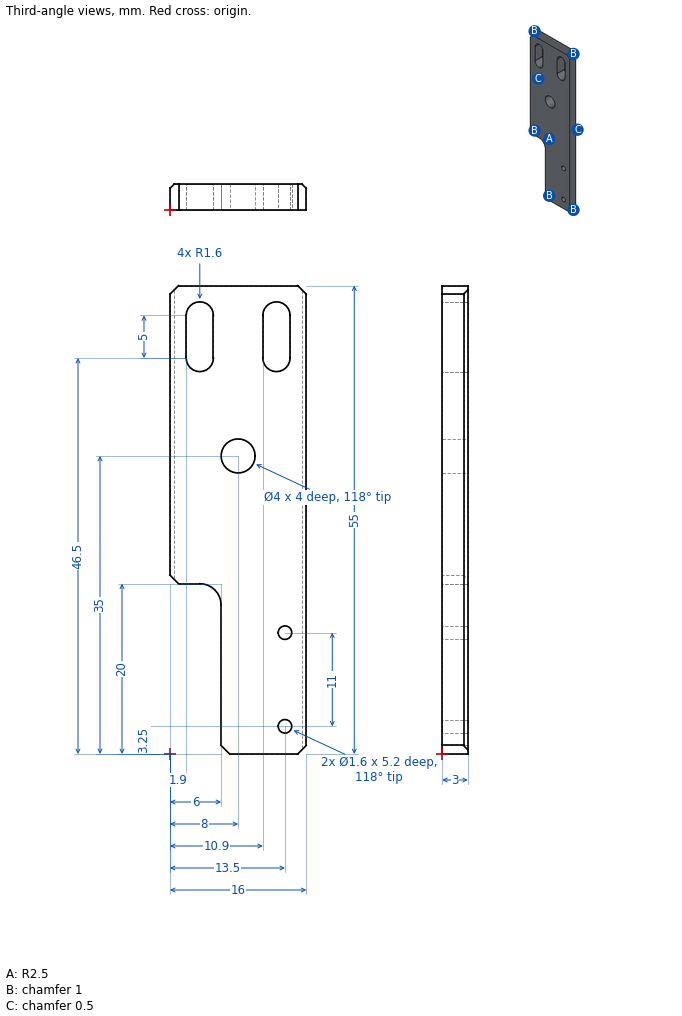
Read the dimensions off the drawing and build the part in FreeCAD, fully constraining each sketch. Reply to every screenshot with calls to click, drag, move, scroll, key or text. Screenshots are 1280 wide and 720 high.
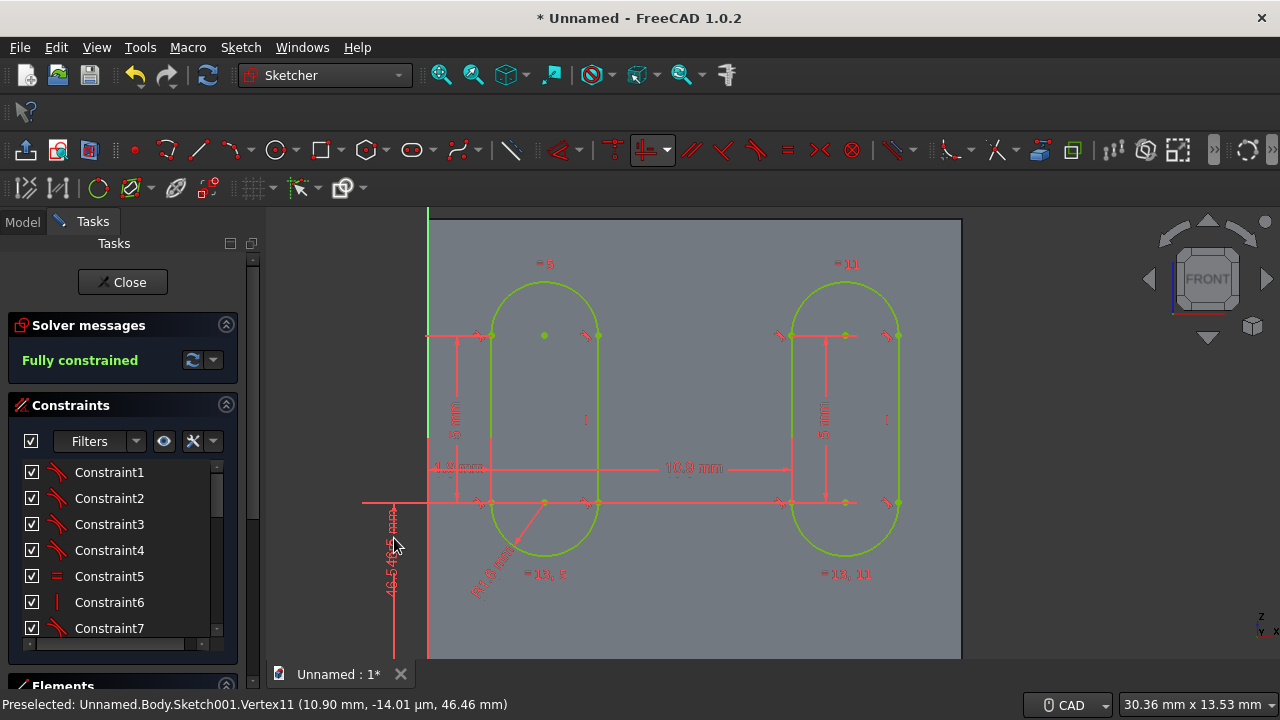
click(123, 282)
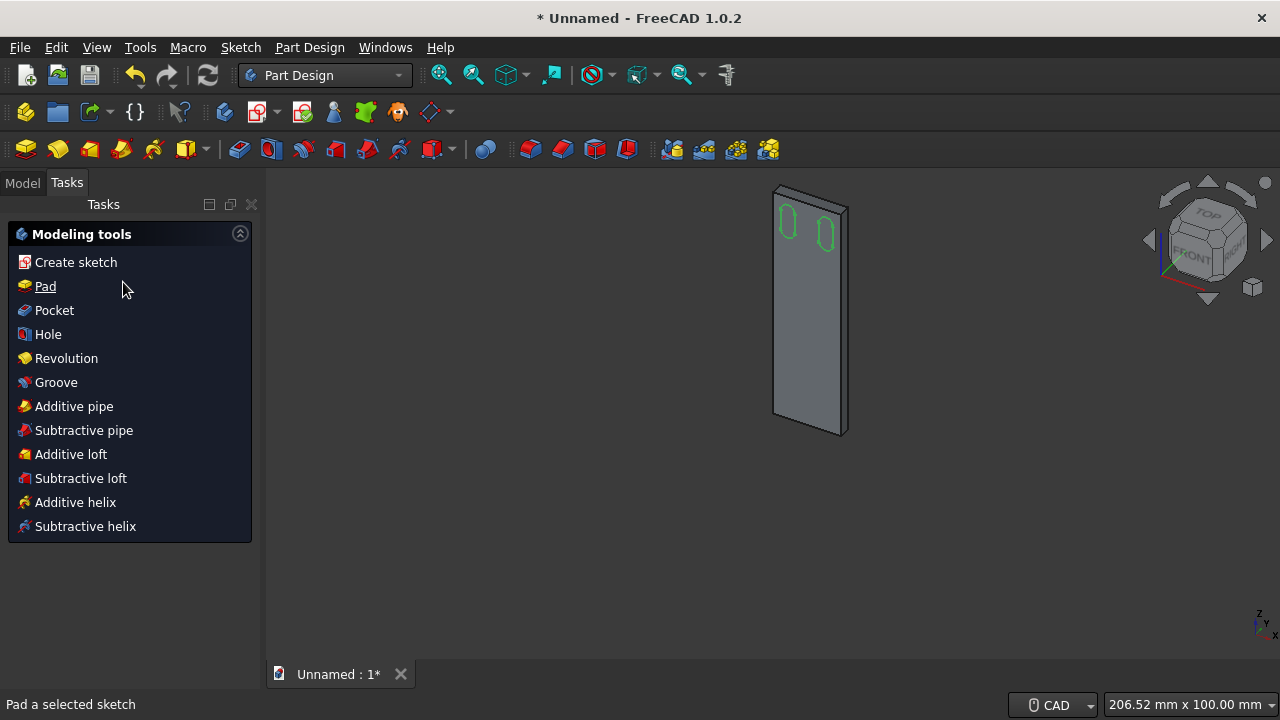
click(240, 150)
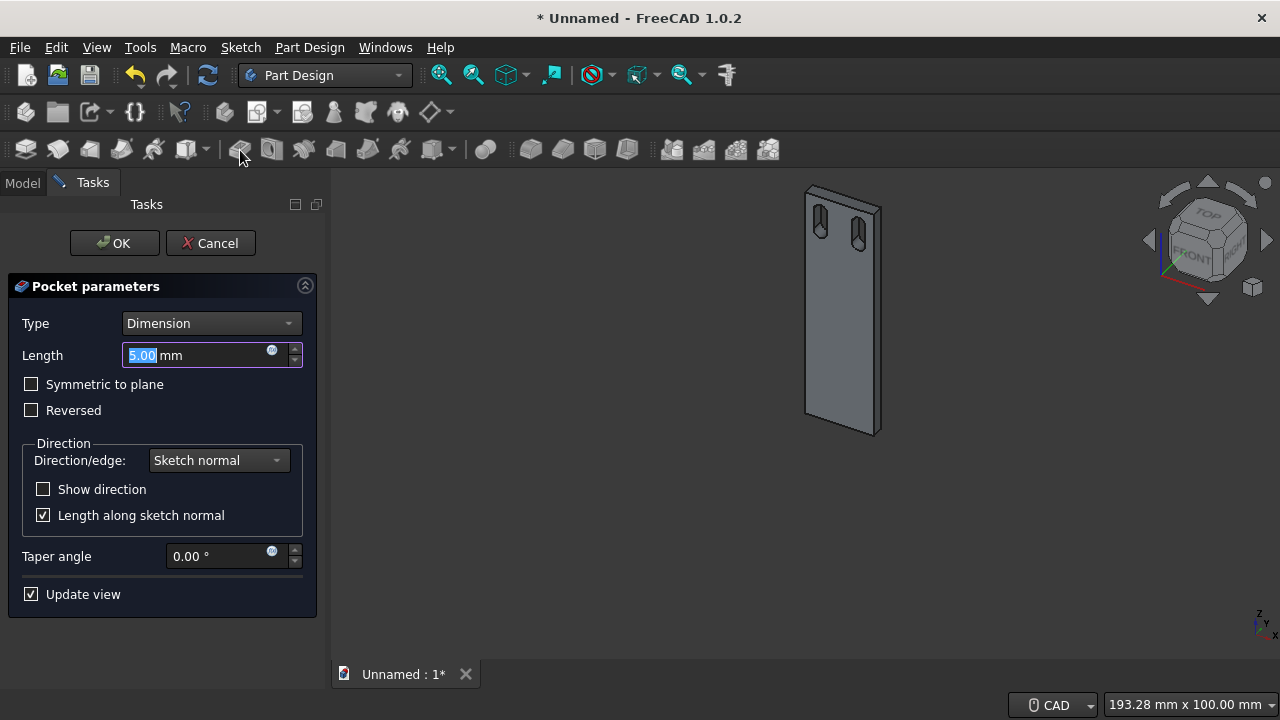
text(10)
key(Tab)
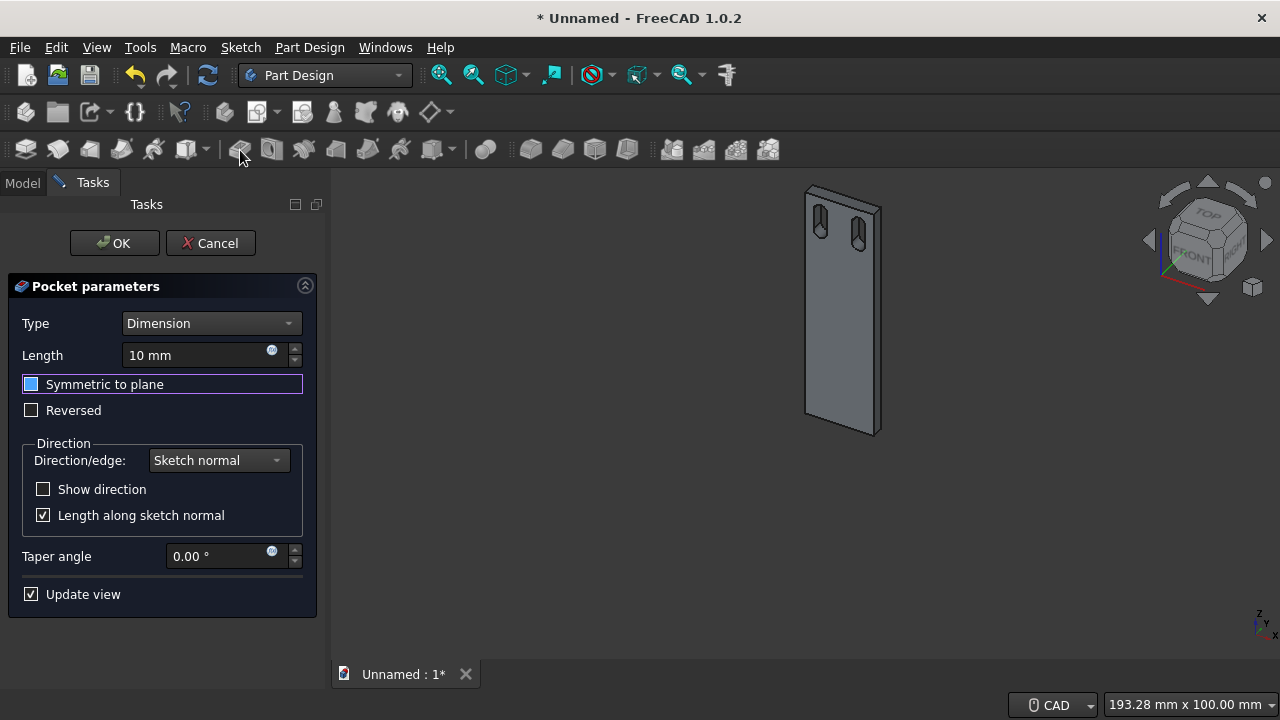
click(115, 243)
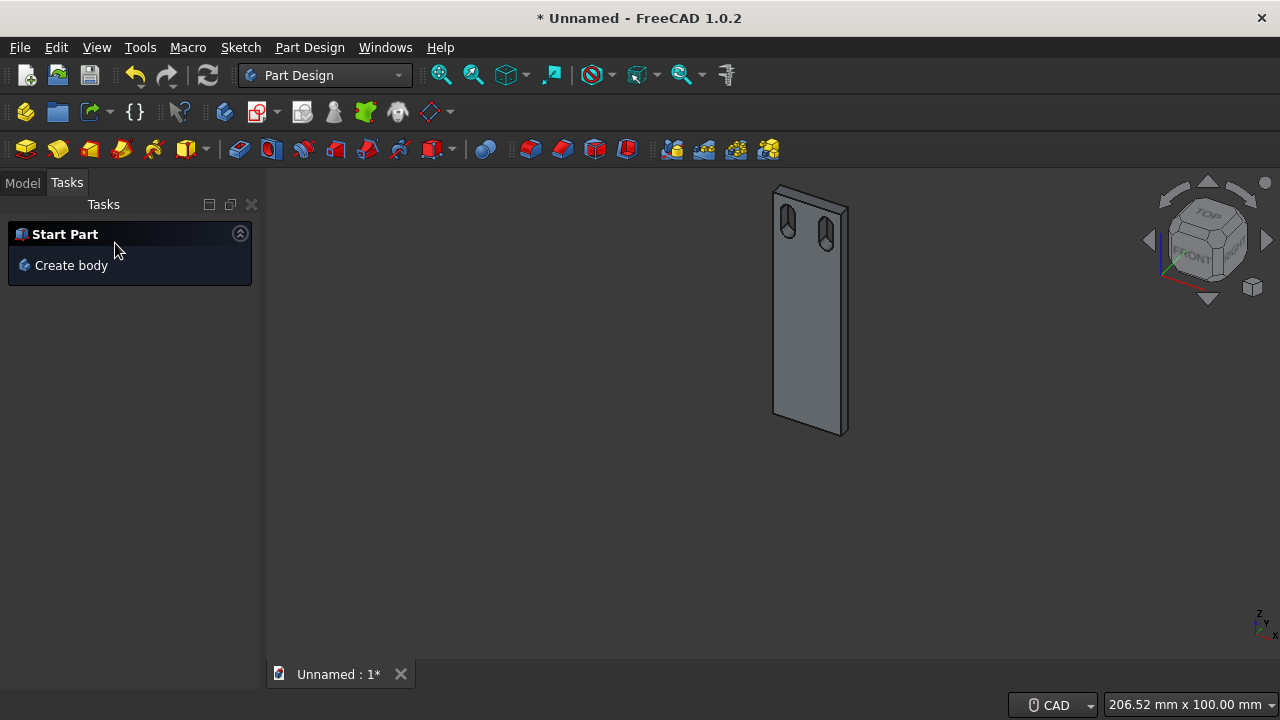
key(4)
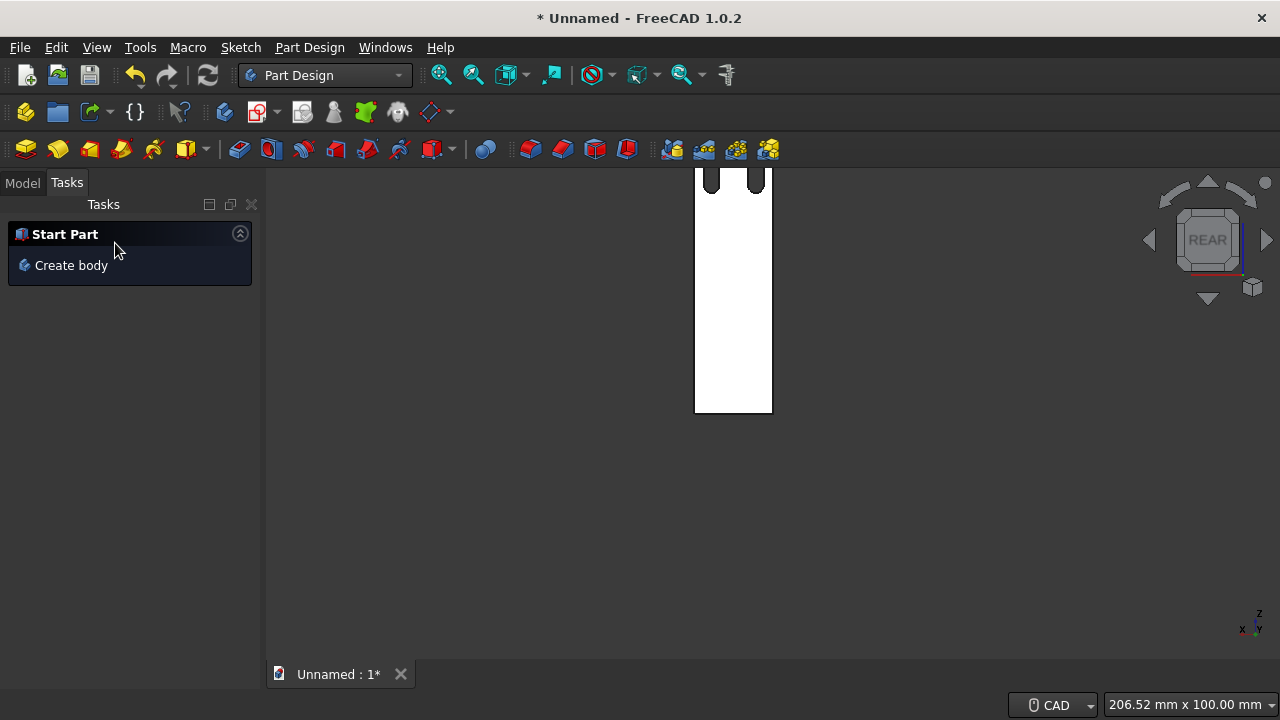
click(442, 76)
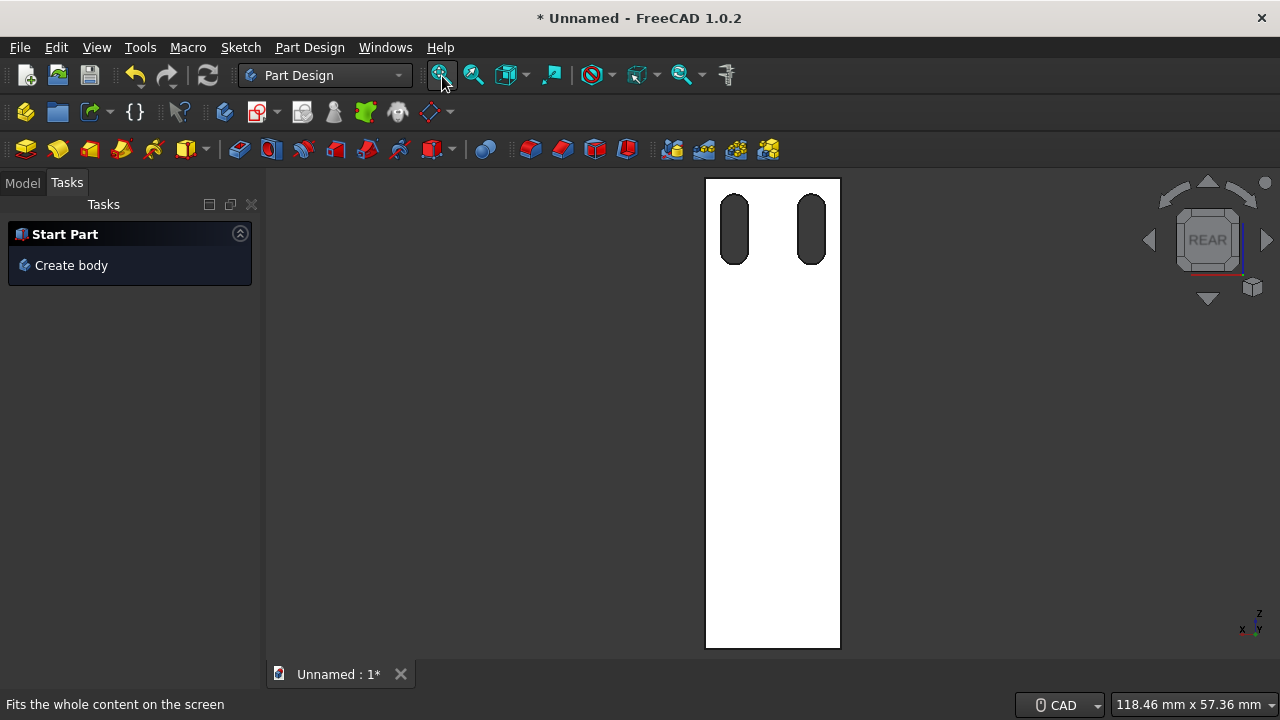
click(773, 345)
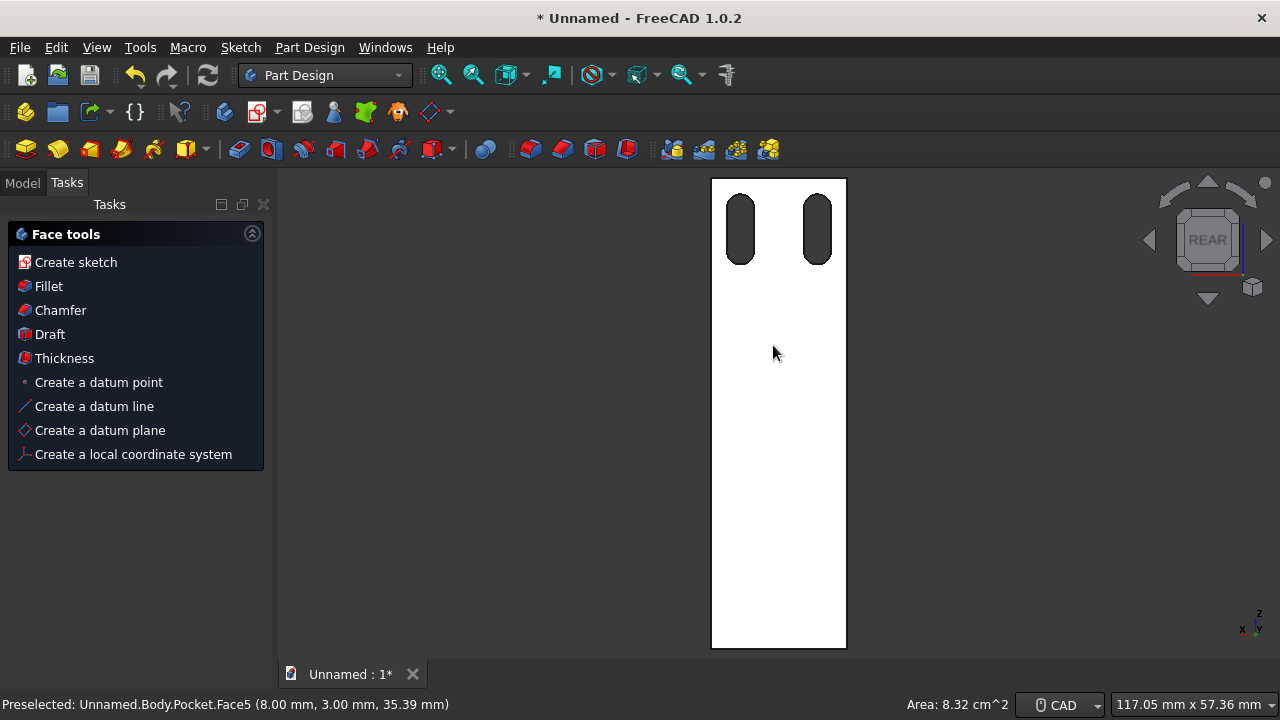
click(258, 112)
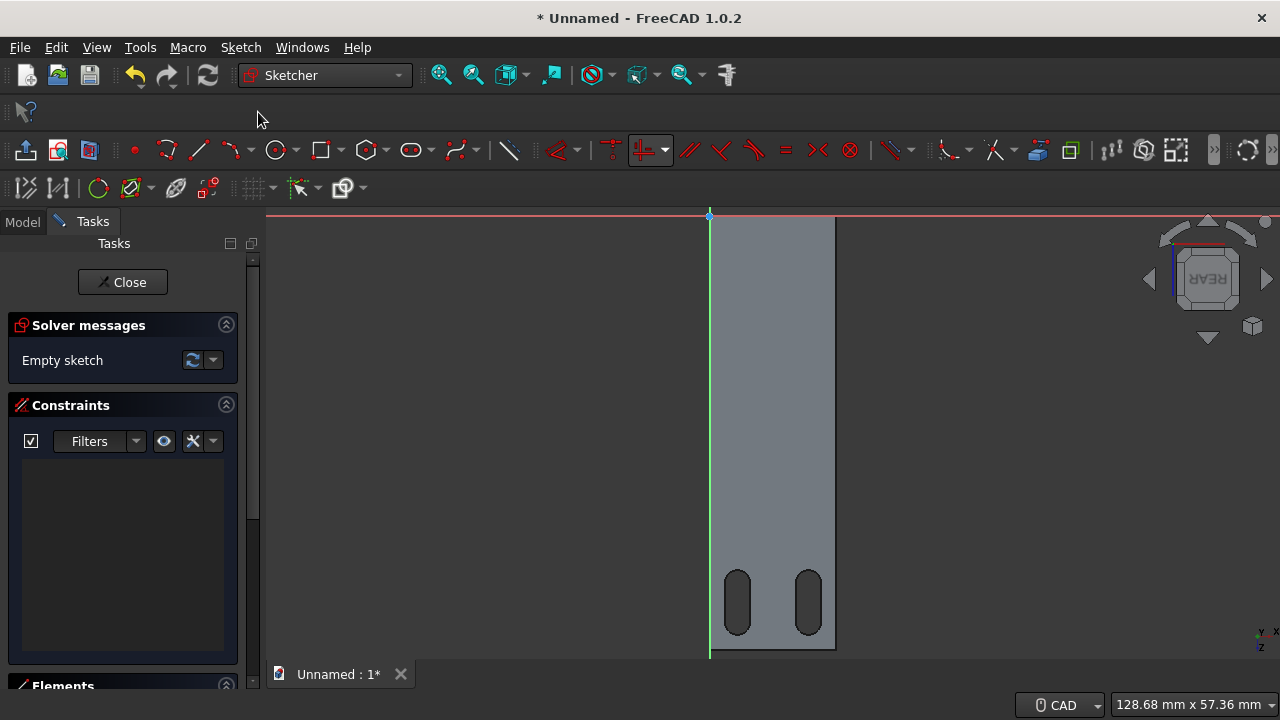
scroll(704, 433, down, 5)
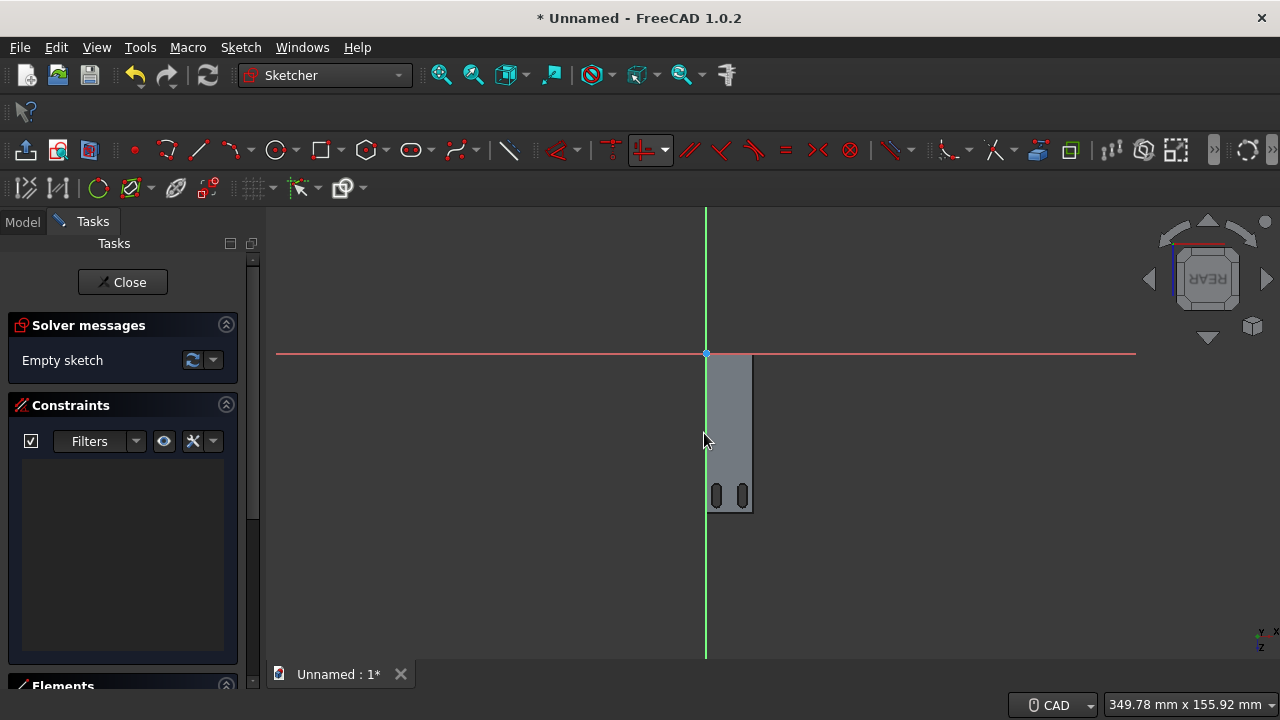
scroll(718, 370, up, 8)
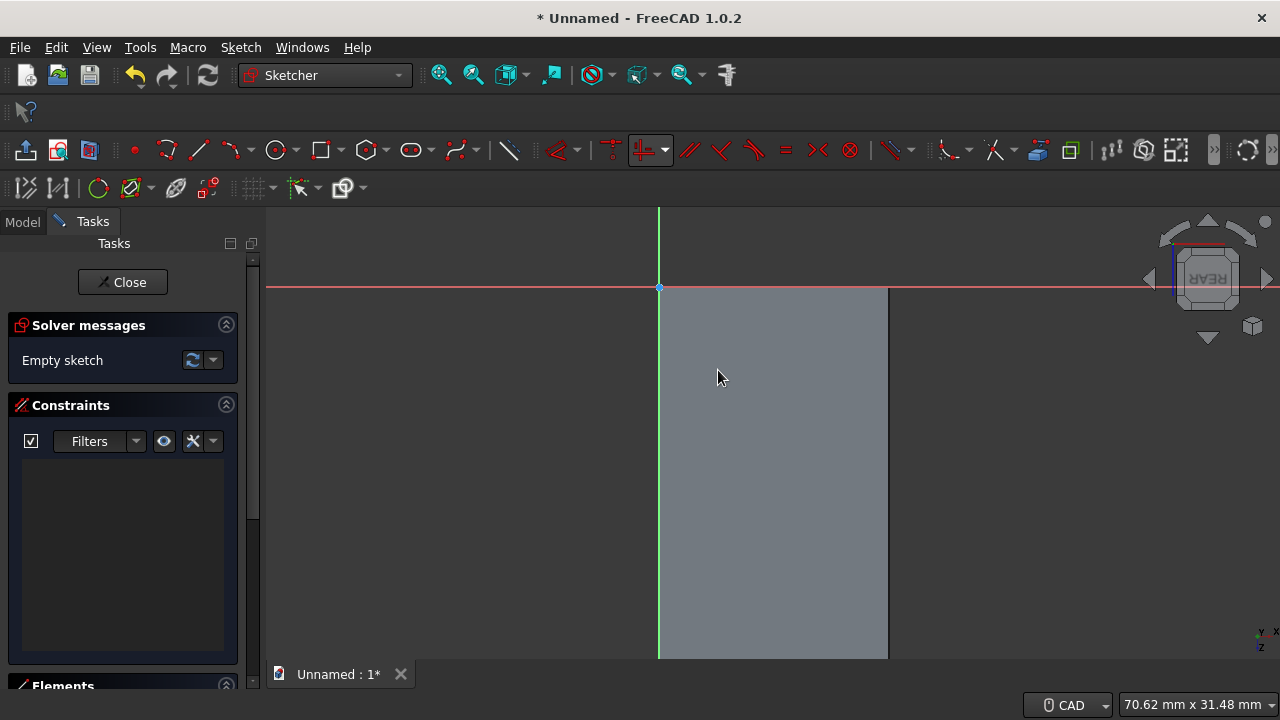
click(322, 150)